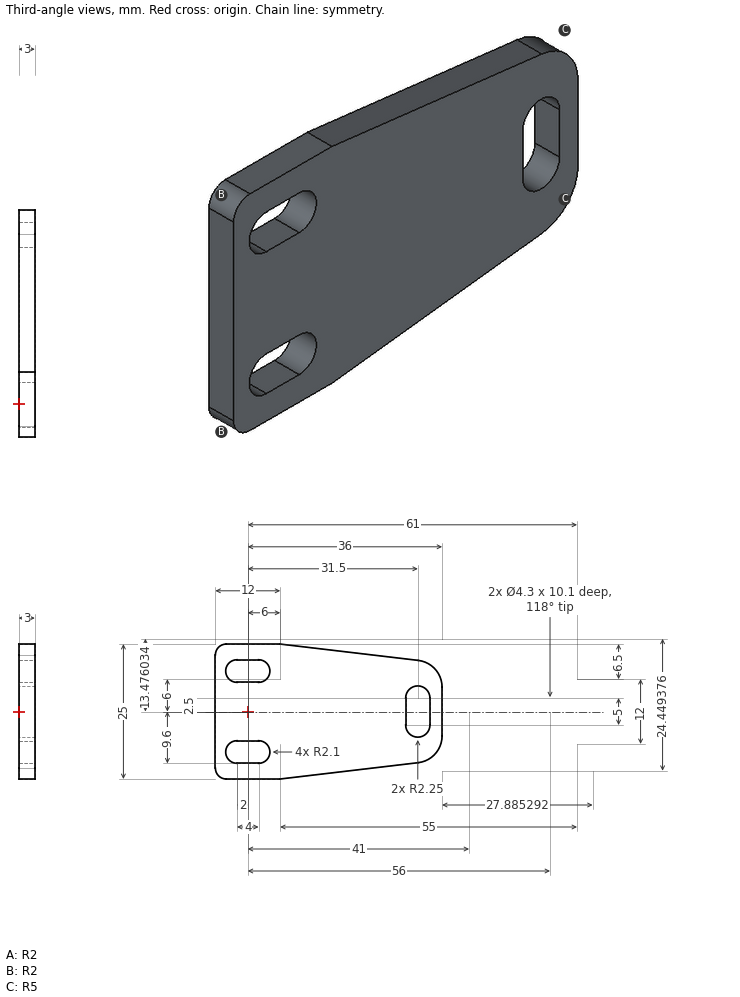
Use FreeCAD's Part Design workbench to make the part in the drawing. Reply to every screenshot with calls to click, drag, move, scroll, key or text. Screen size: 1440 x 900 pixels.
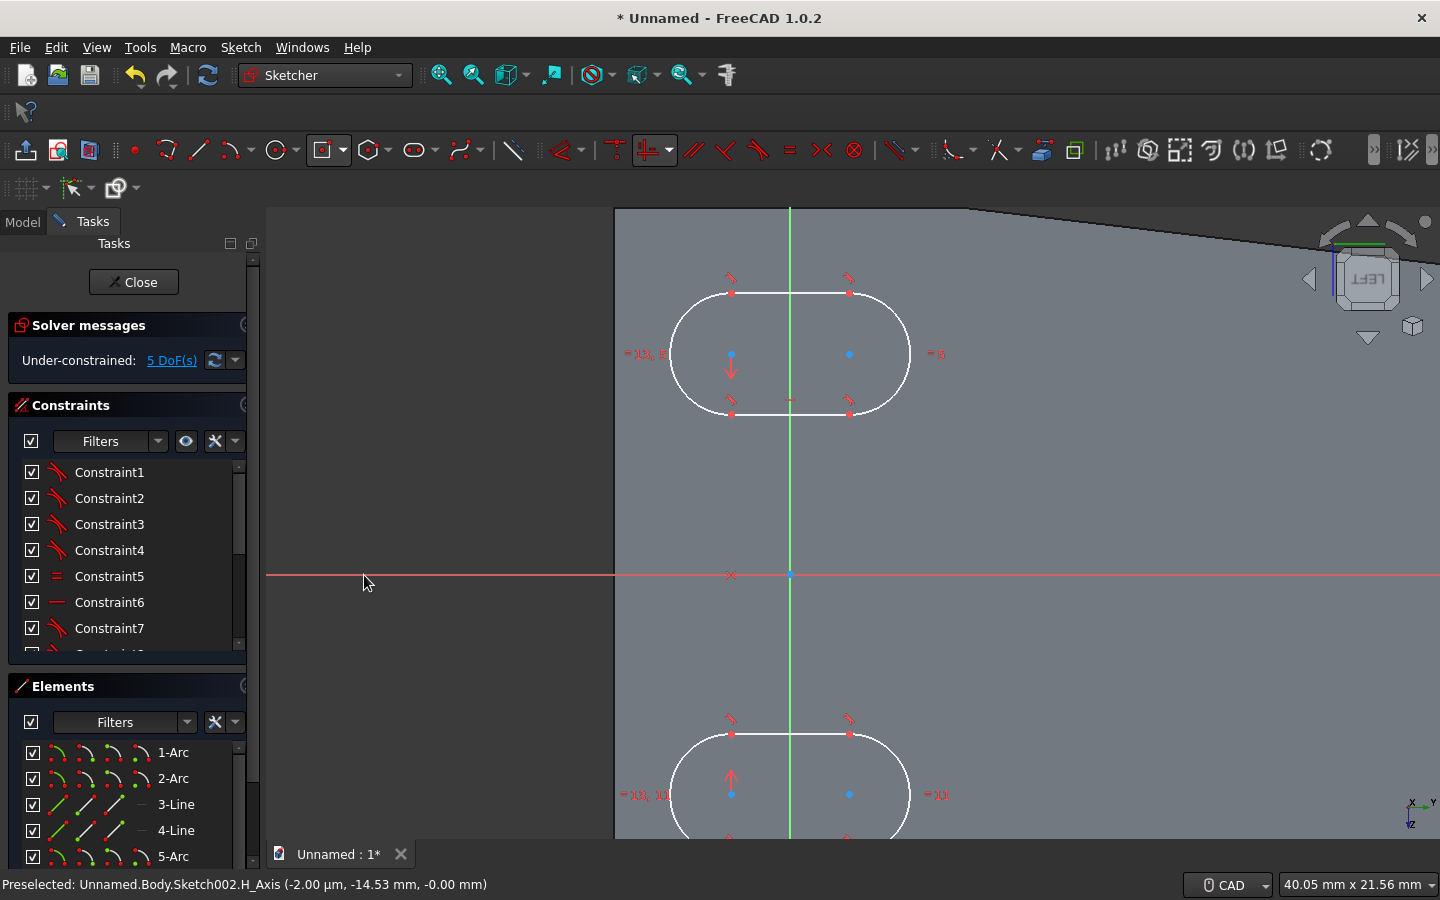
click(682, 318)
click(656, 299)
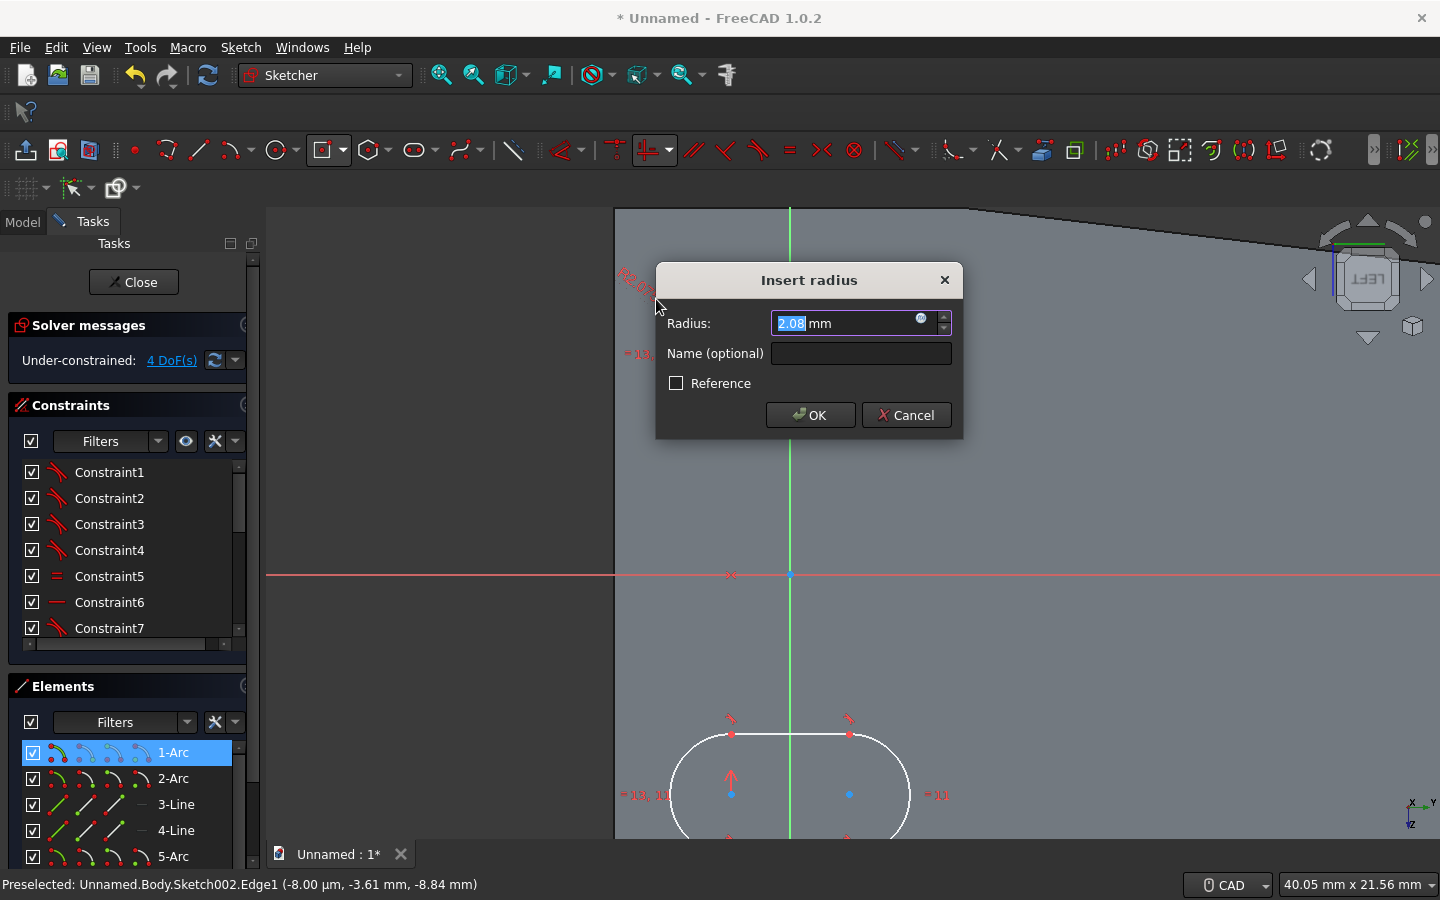
text(2.1)
key(Return)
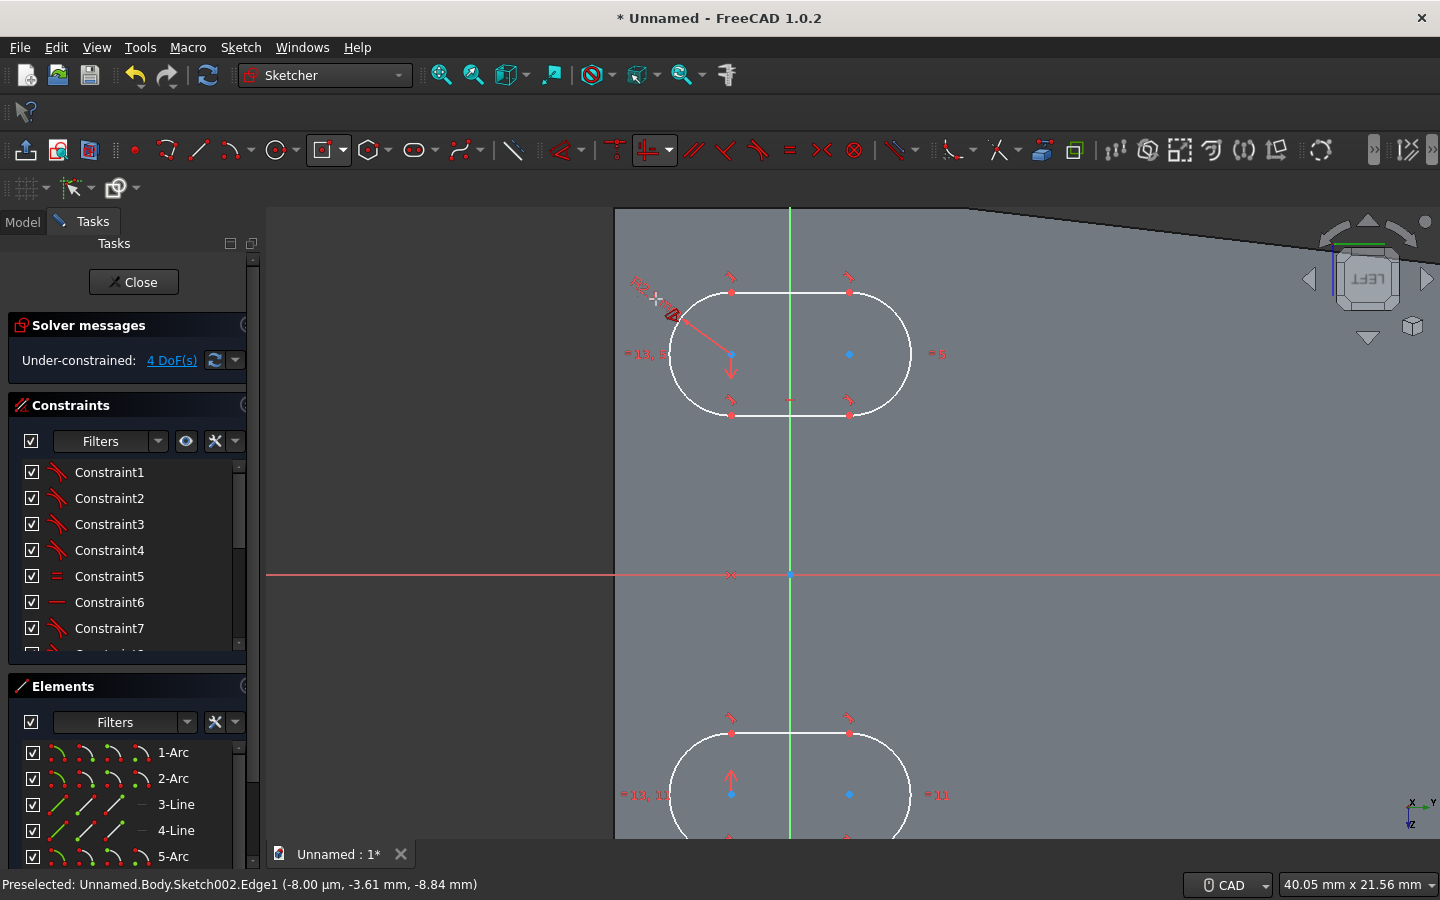
click(767, 293)
click(763, 259)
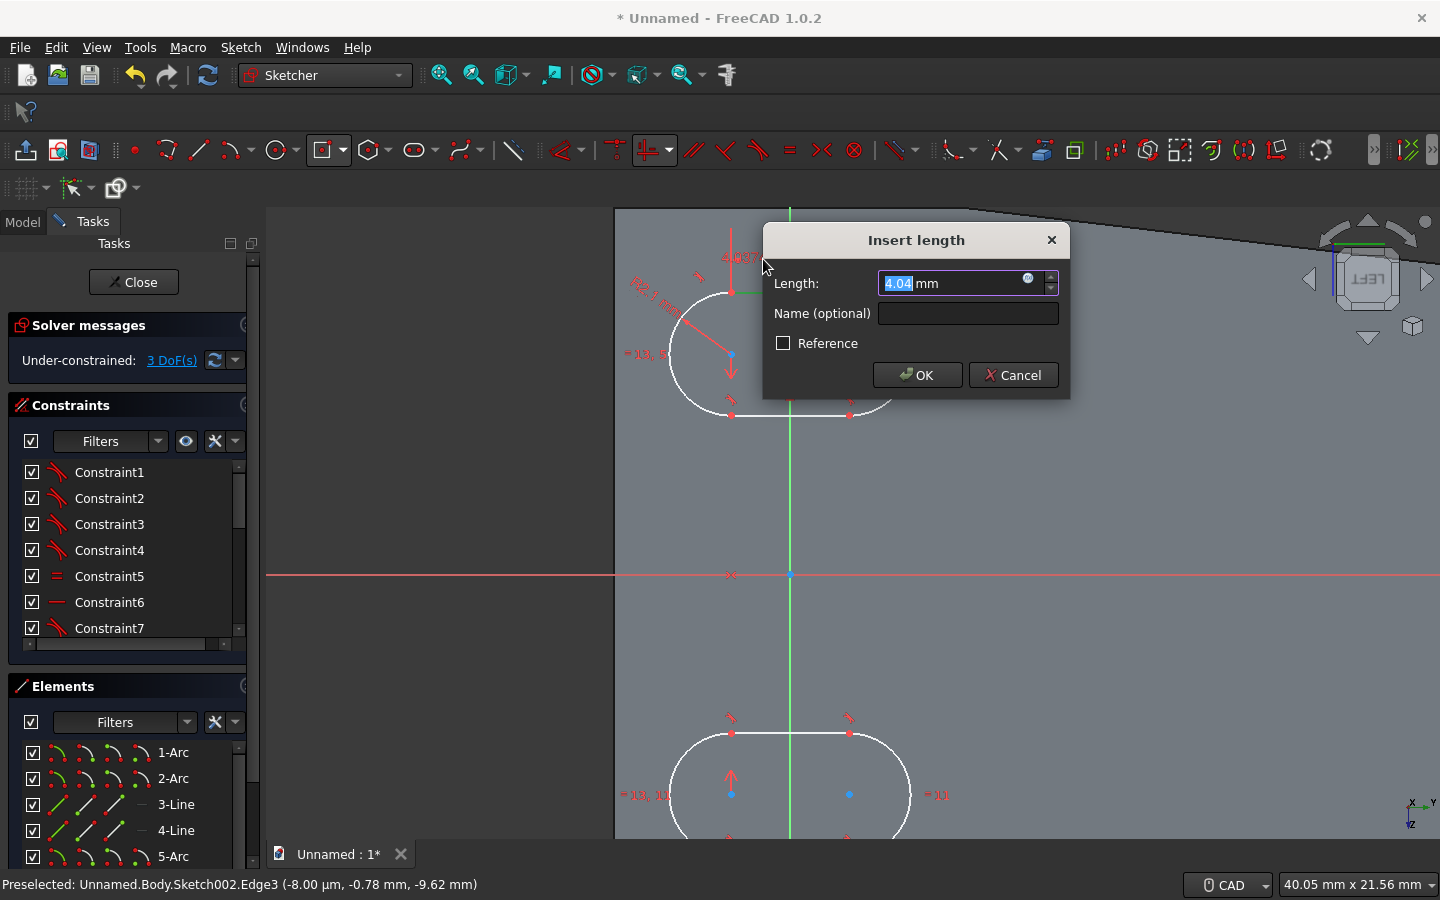
text(4)
key(Return)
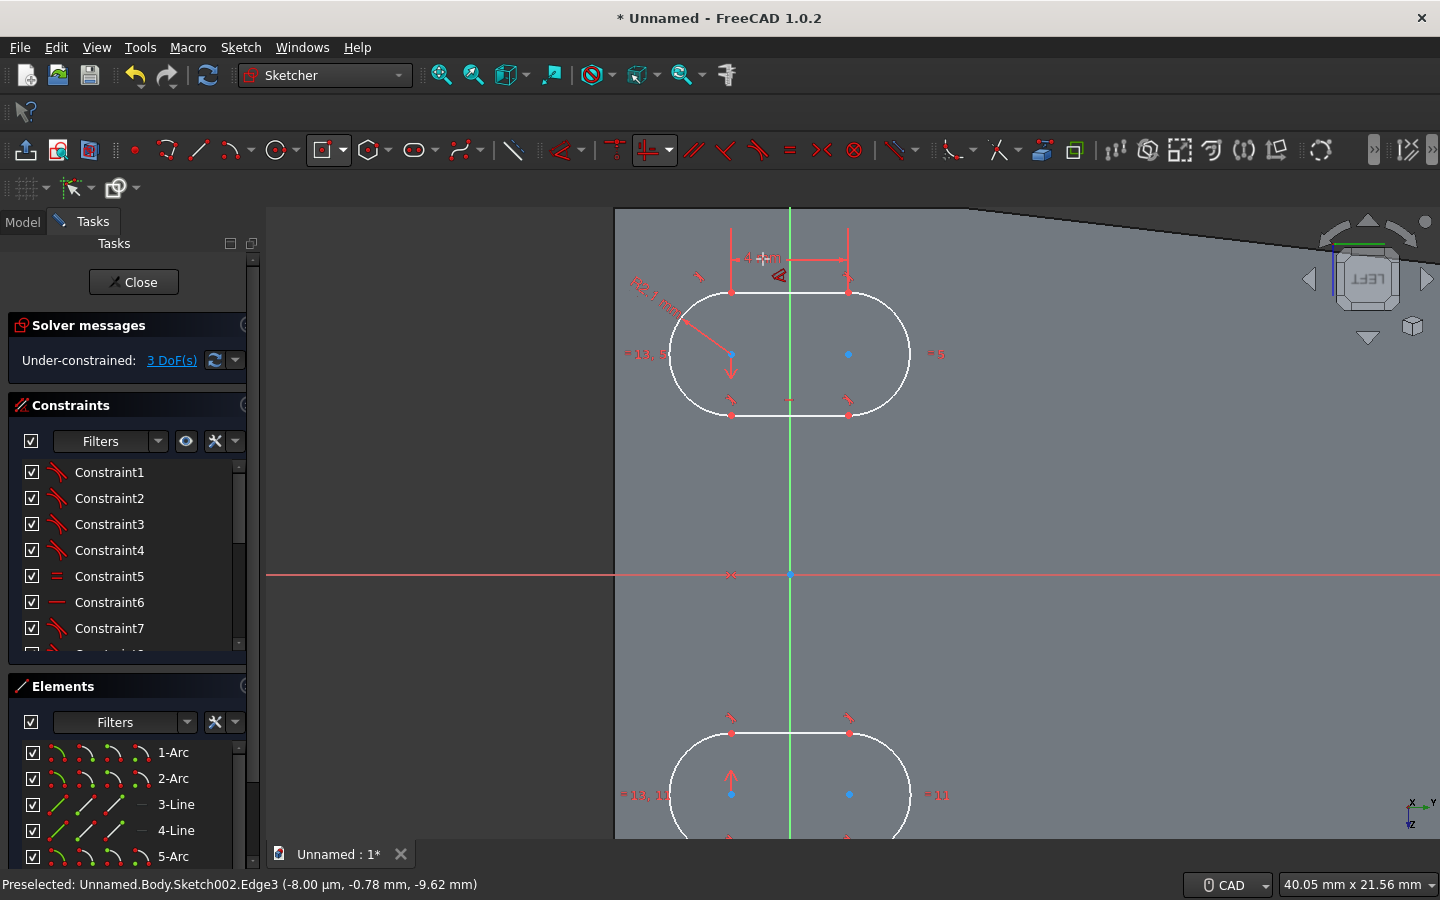
click(766, 733)
click(763, 767)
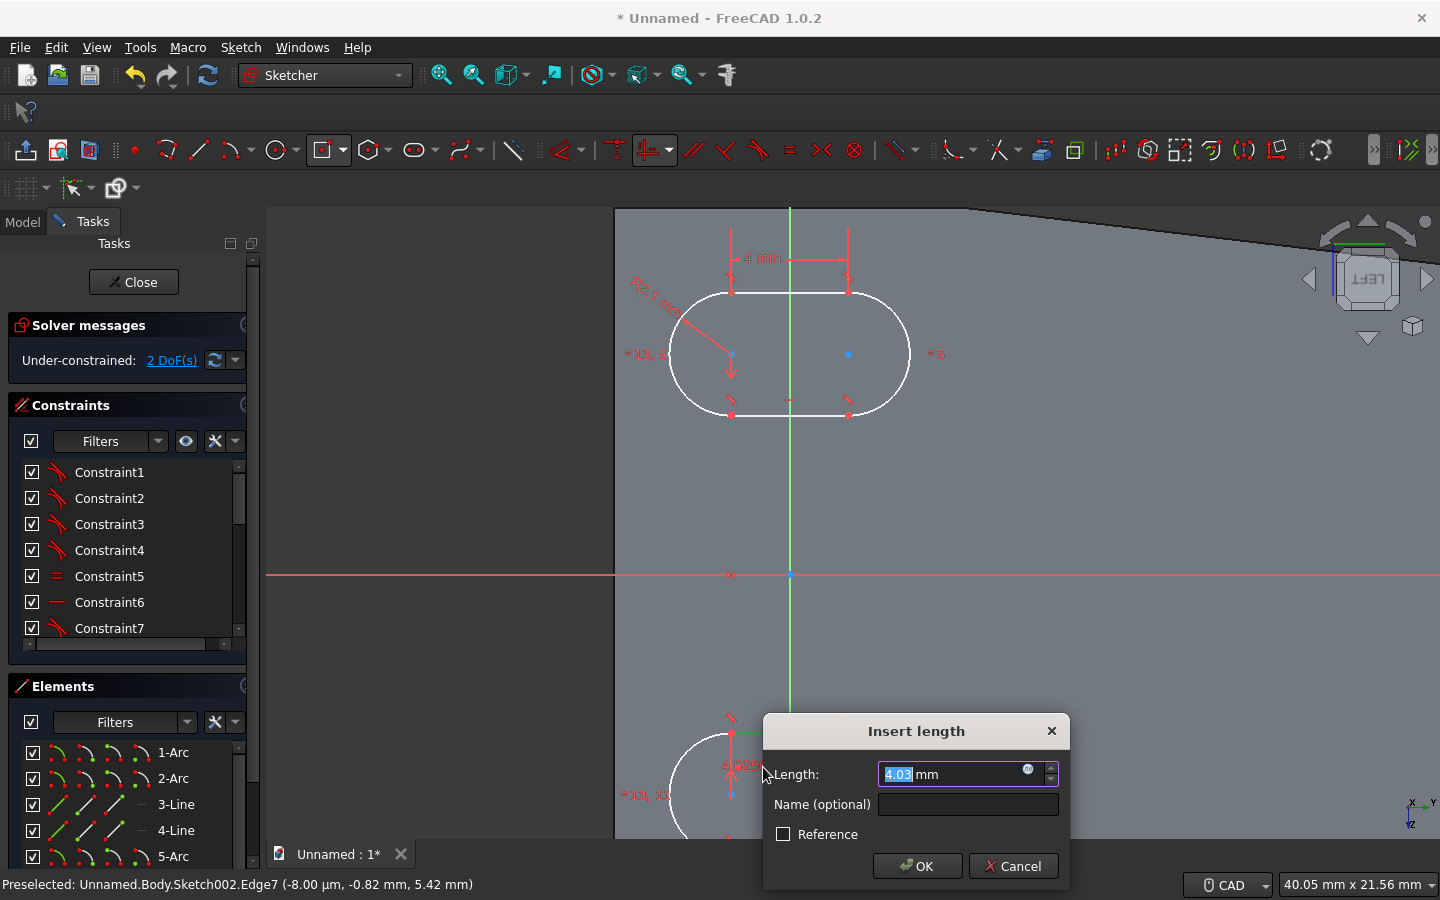
text(4)
key(Return)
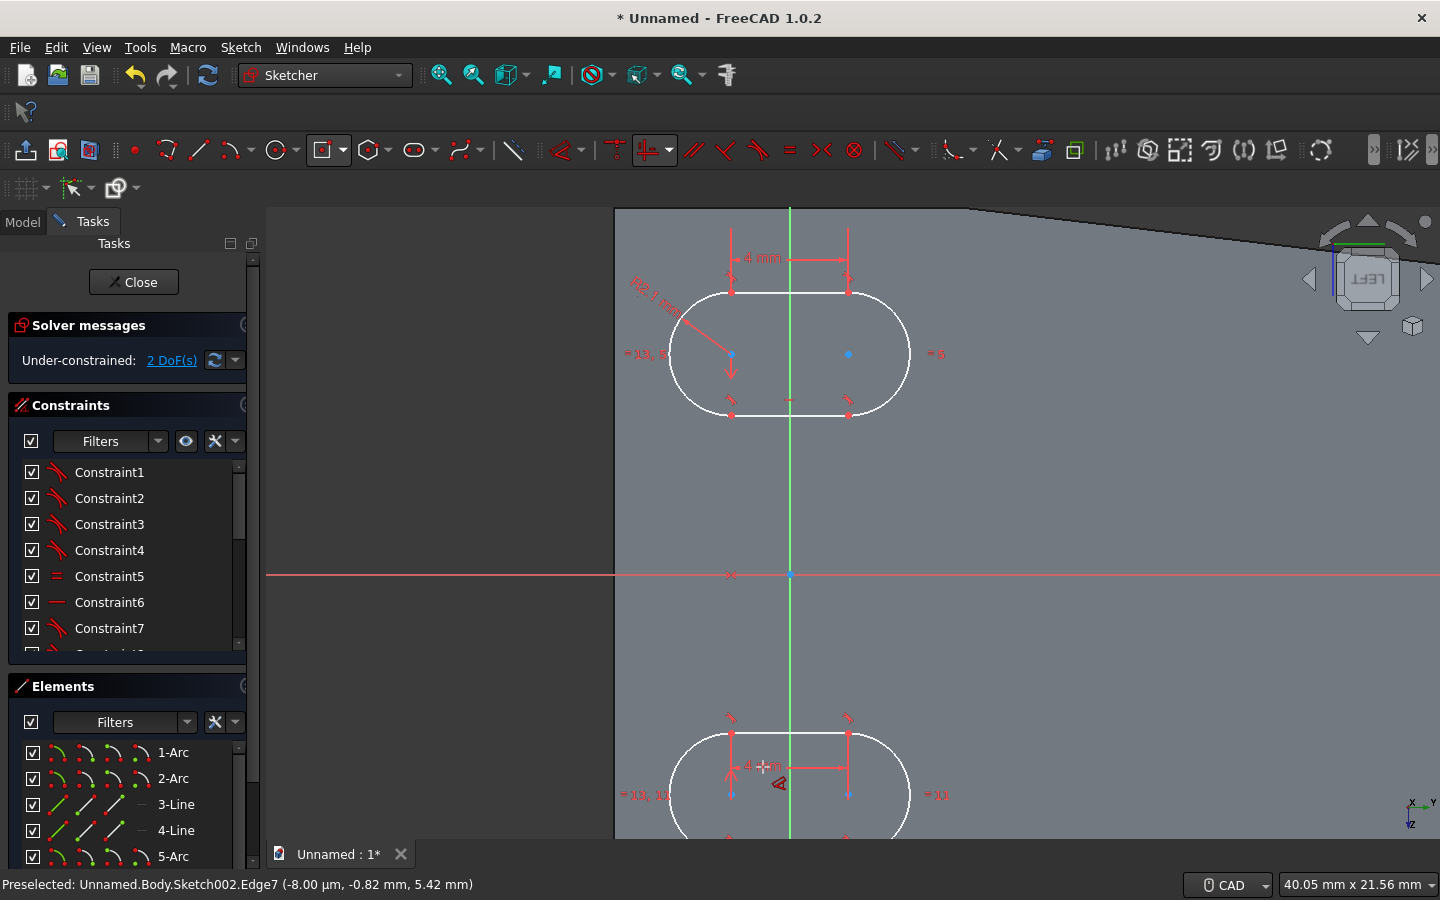
click(731, 293)
click(761, 609)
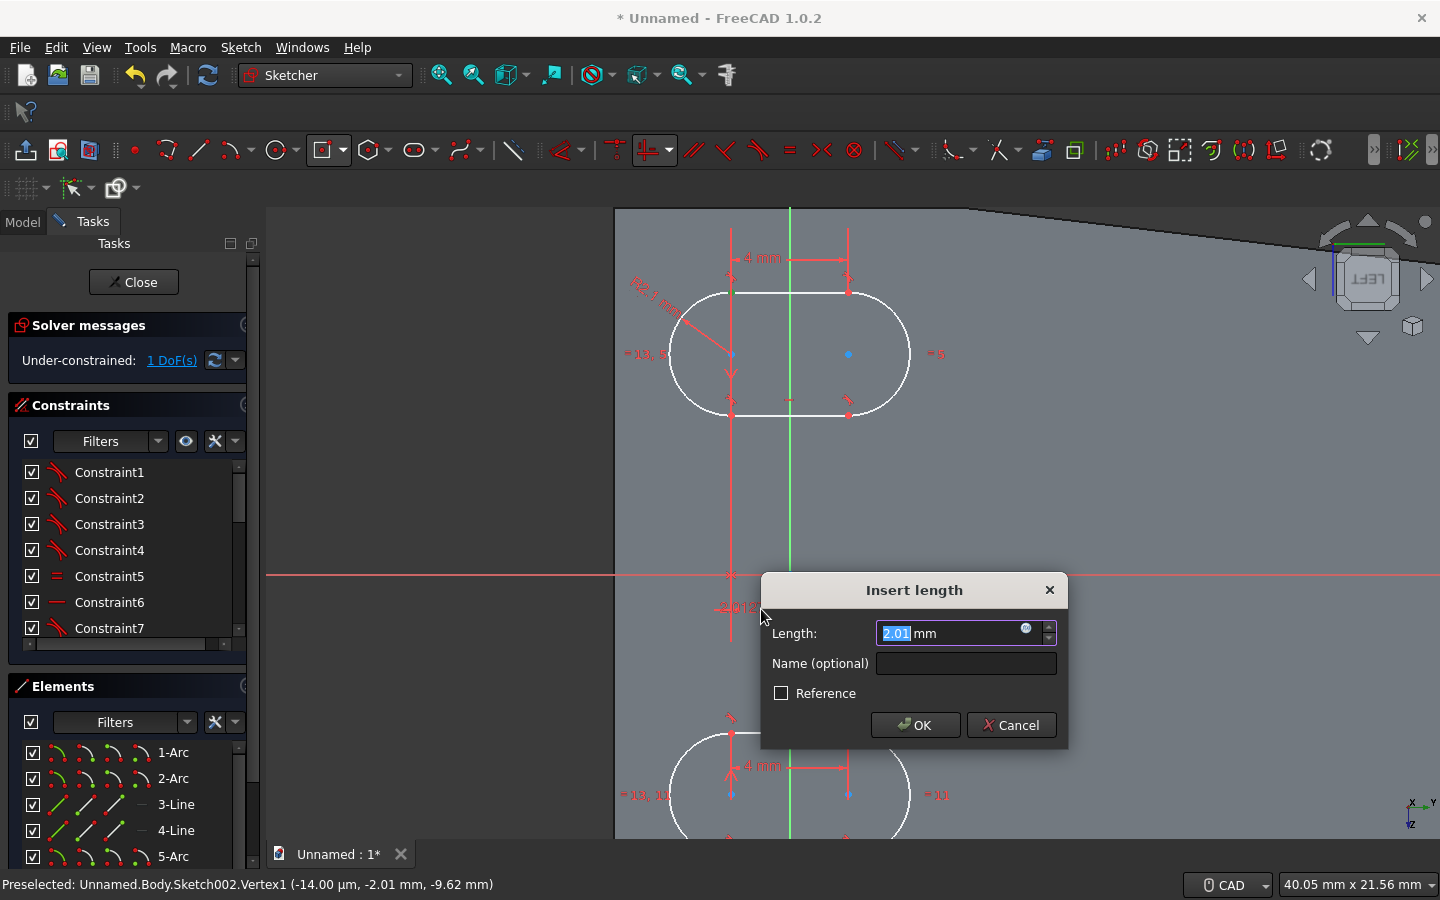
text(2)
key(Return)